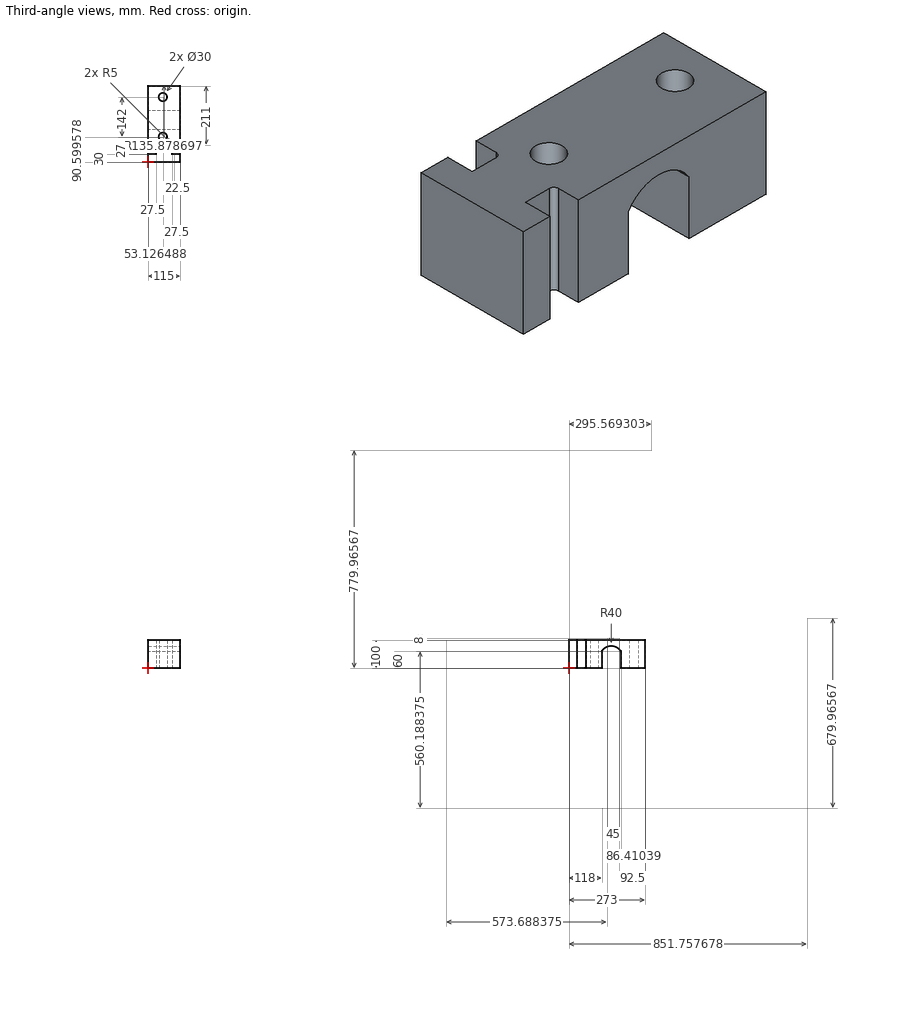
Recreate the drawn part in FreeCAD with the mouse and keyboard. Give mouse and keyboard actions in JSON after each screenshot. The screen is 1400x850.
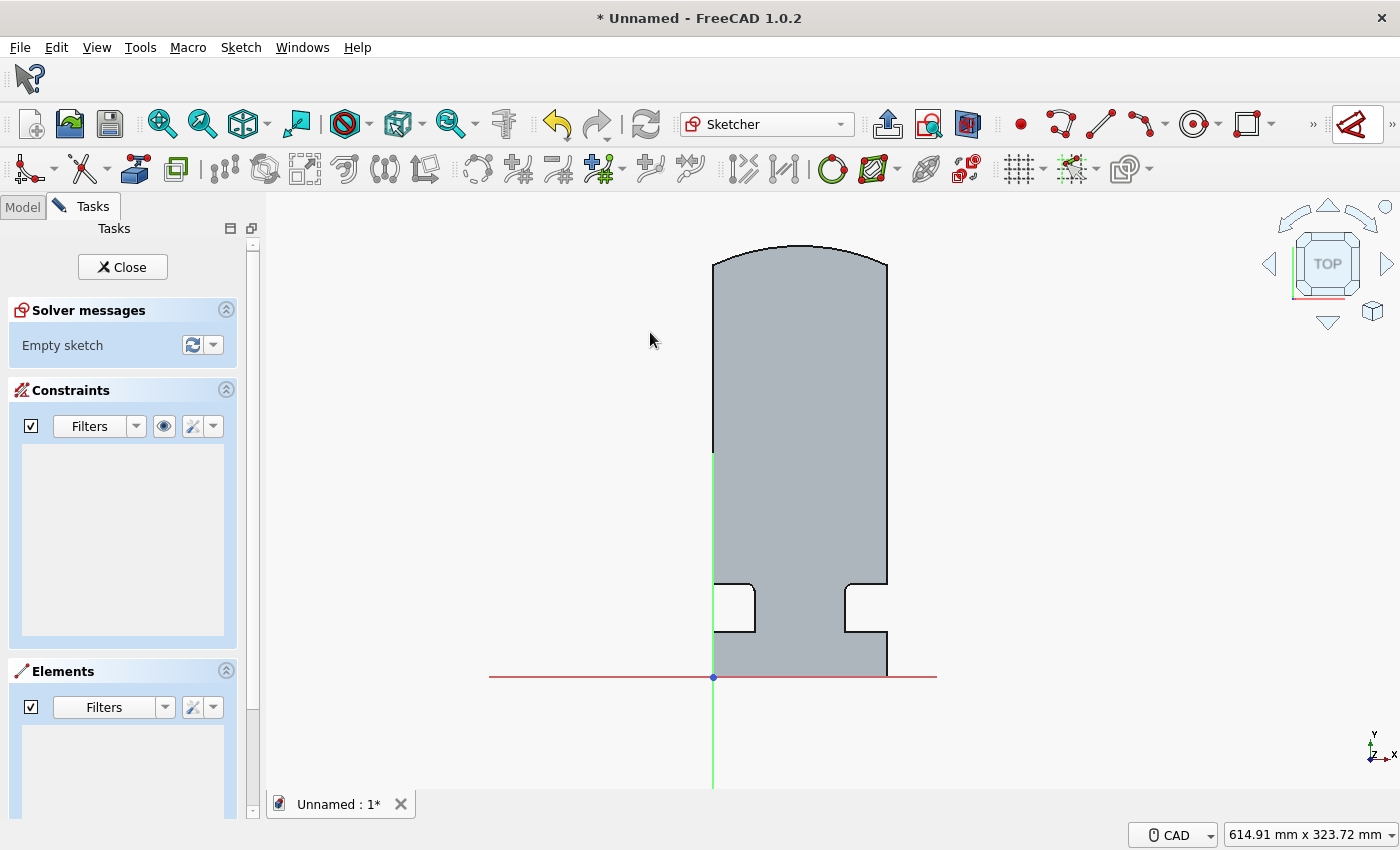
{"action": "key", "text": "g c"}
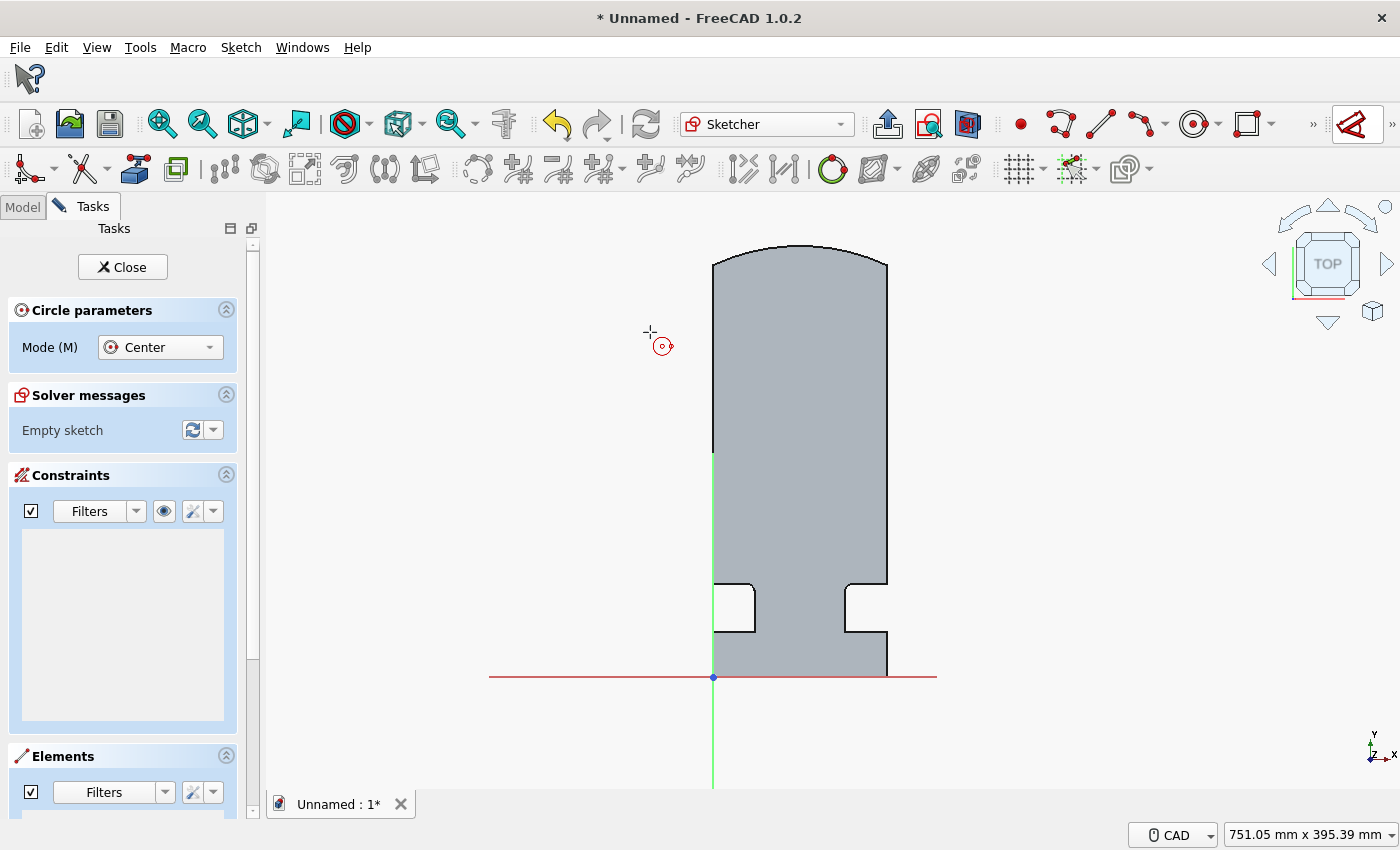
{"action": "left_click", "coordinate": [793, 326]}
{"action": "mouse_move", "coordinate": [809, 310]}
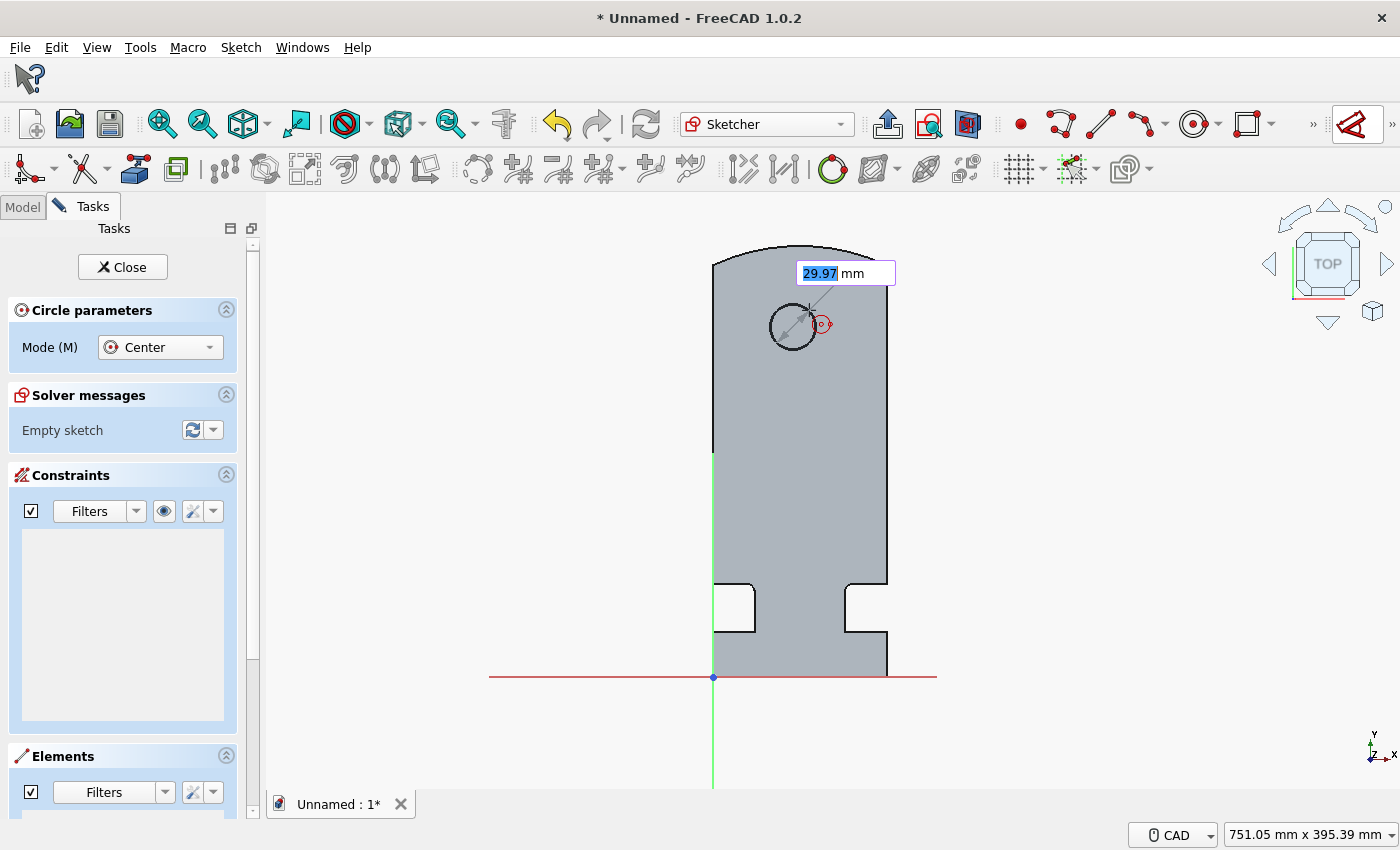
{"action": "type", "text": "30"}
{"action": "key", "text": "Return"}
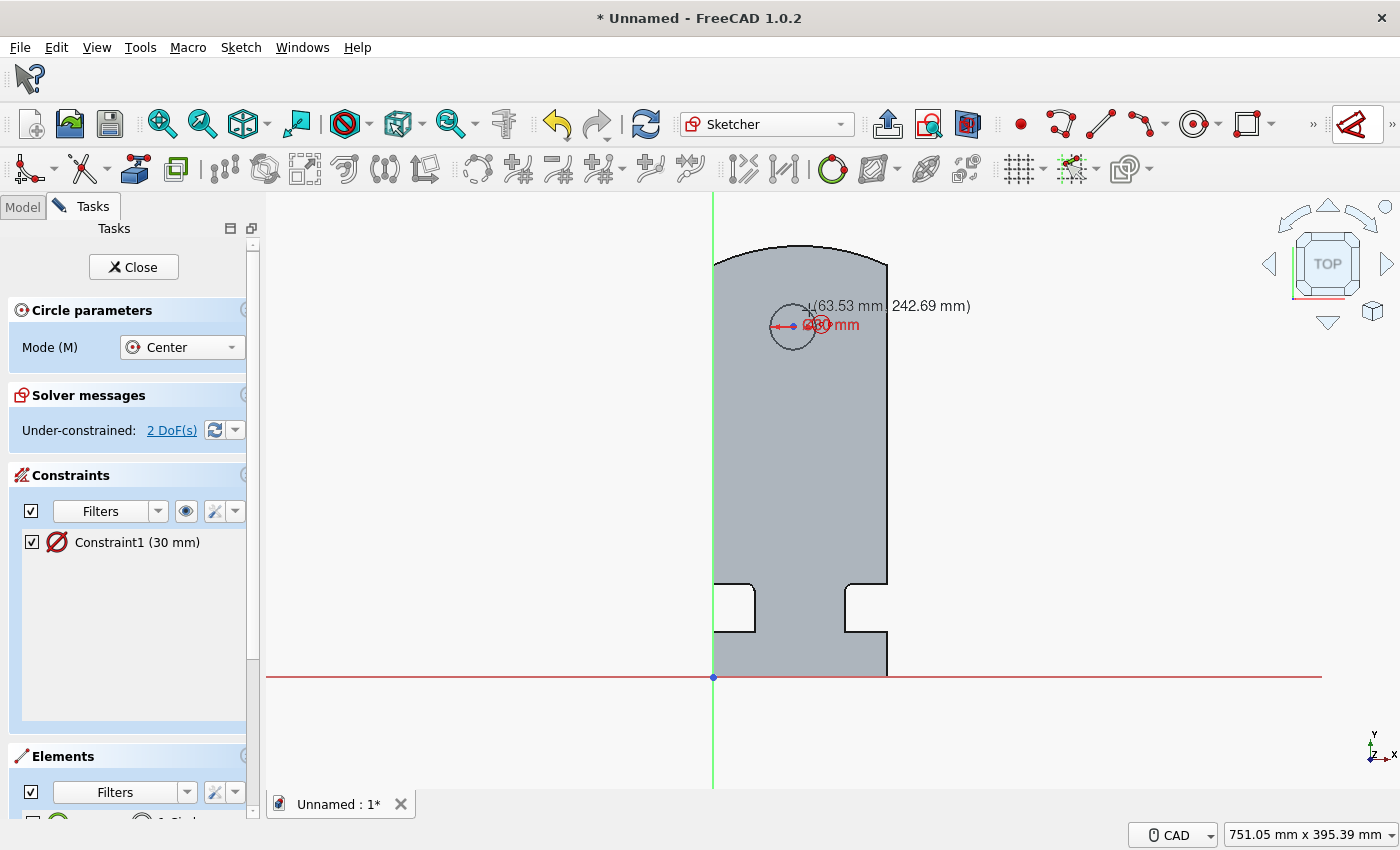
{"action": "left_click", "coordinate": [793, 541]}
{"action": "mouse_move", "coordinate": [809, 525]}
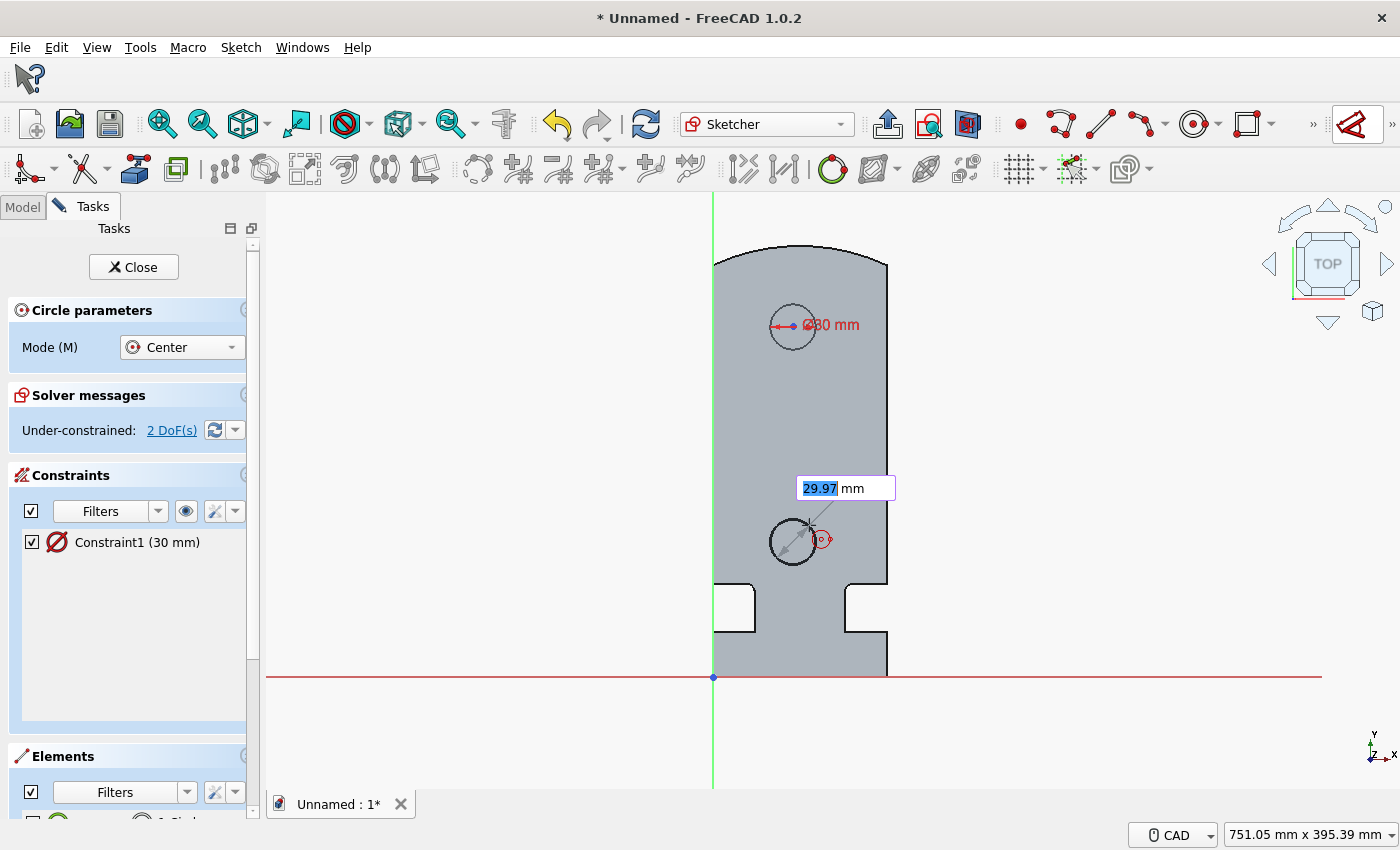
{"action": "type", "text": "30"}
{"action": "key", "text": "Return"}
{"action": "key", "text": "Escape"}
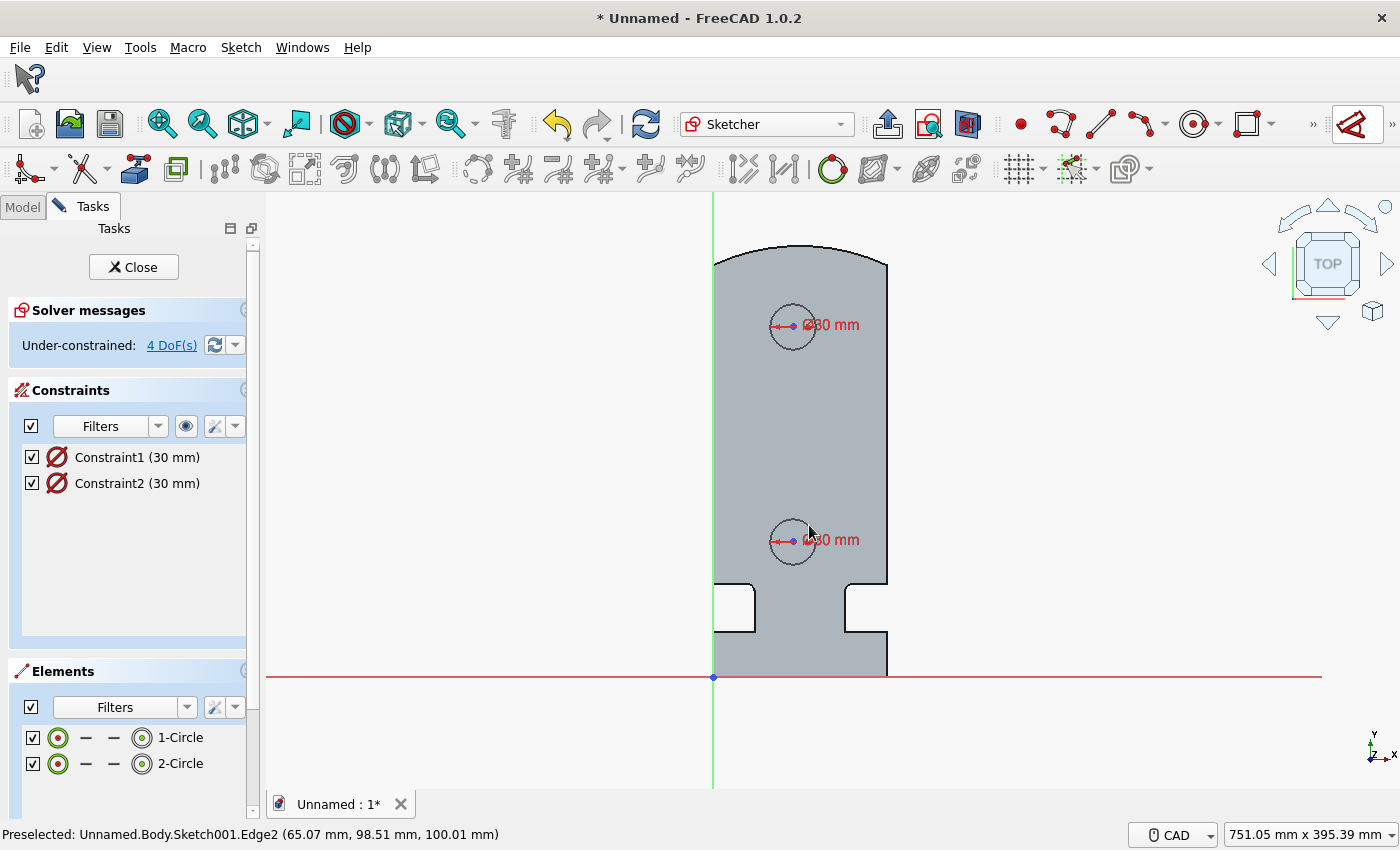
{"action": "left_click", "coordinate": [793, 327]}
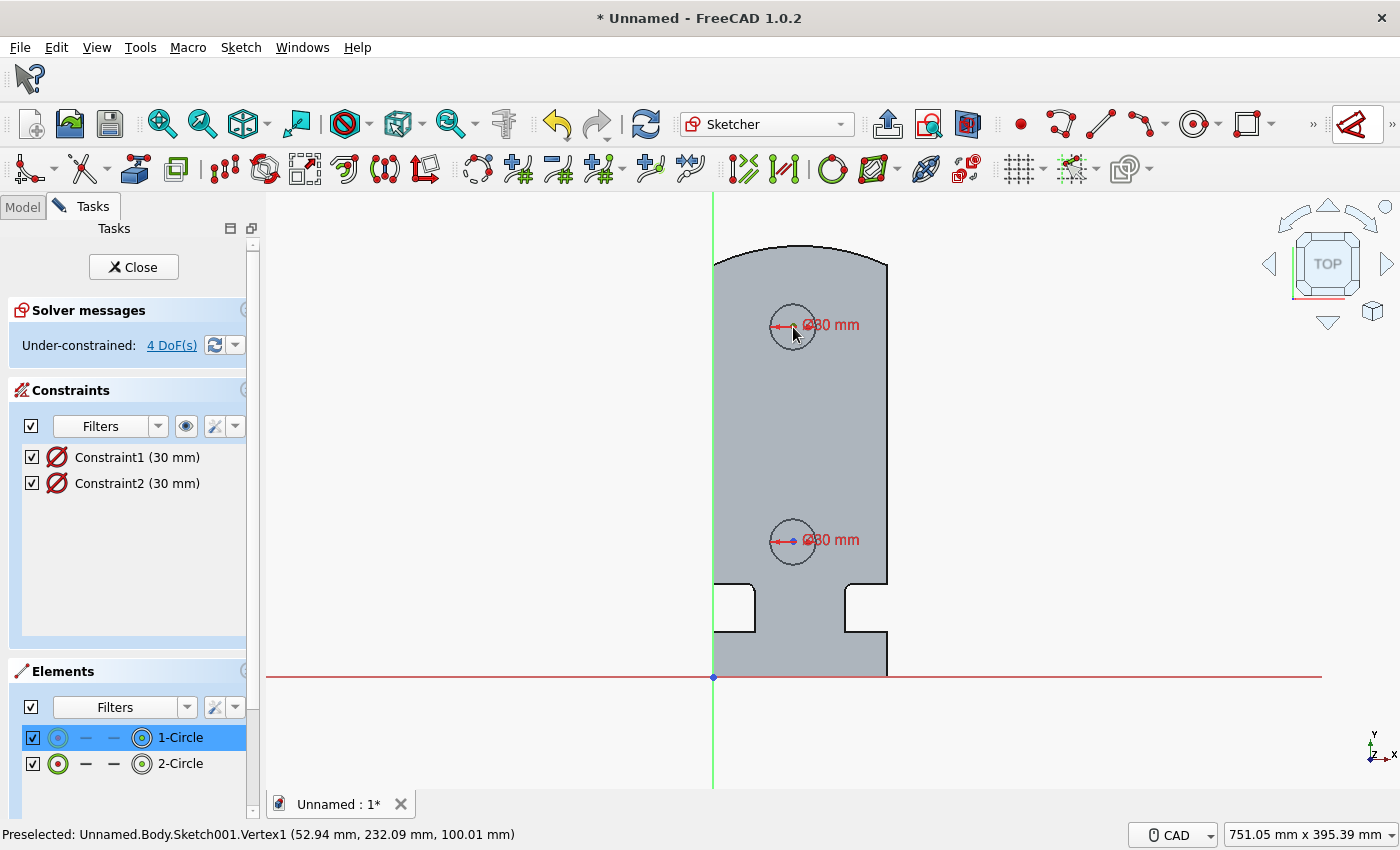
{"action": "left_click", "coordinate": [793, 542]}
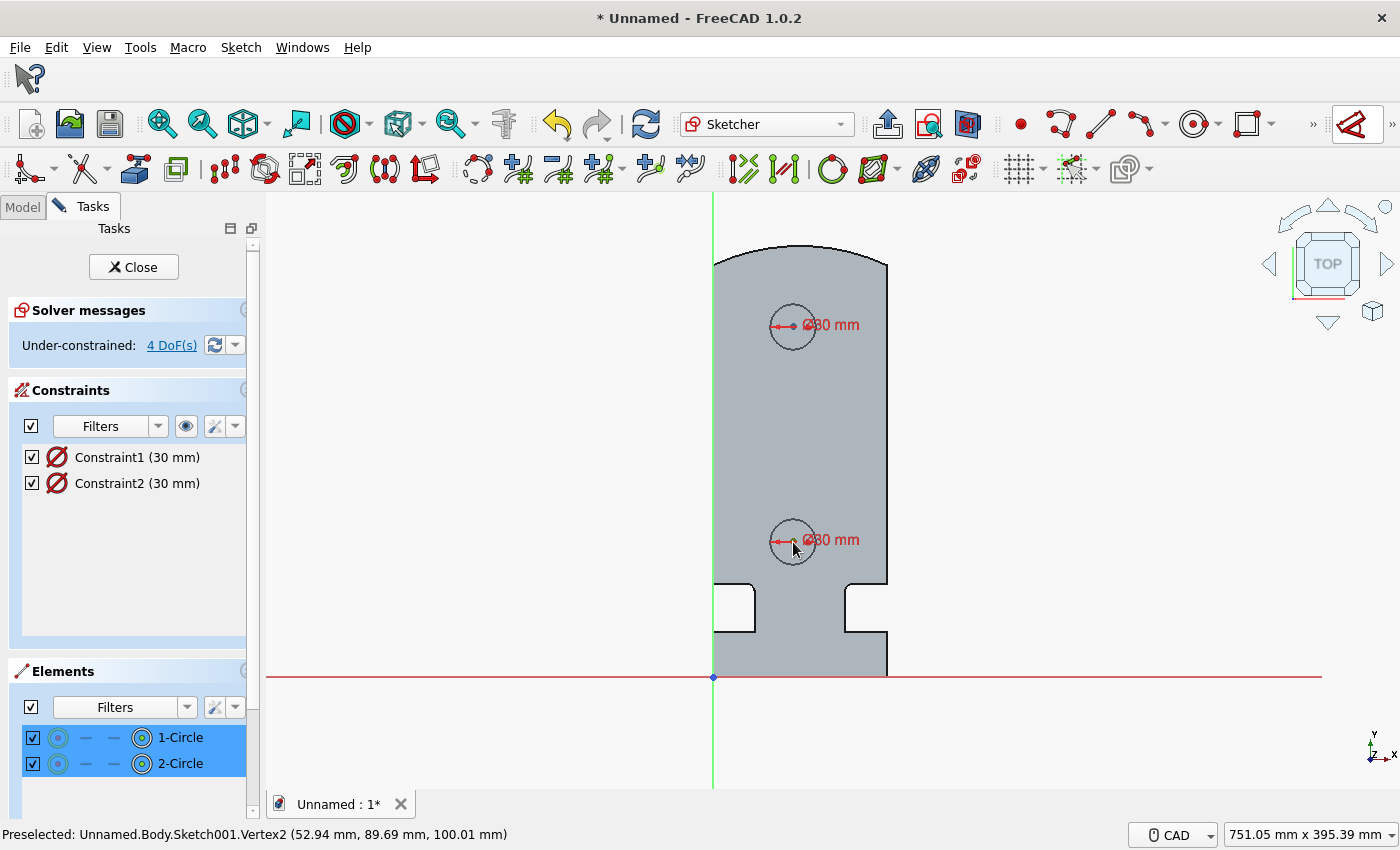
{"action": "key", "text": "v"}